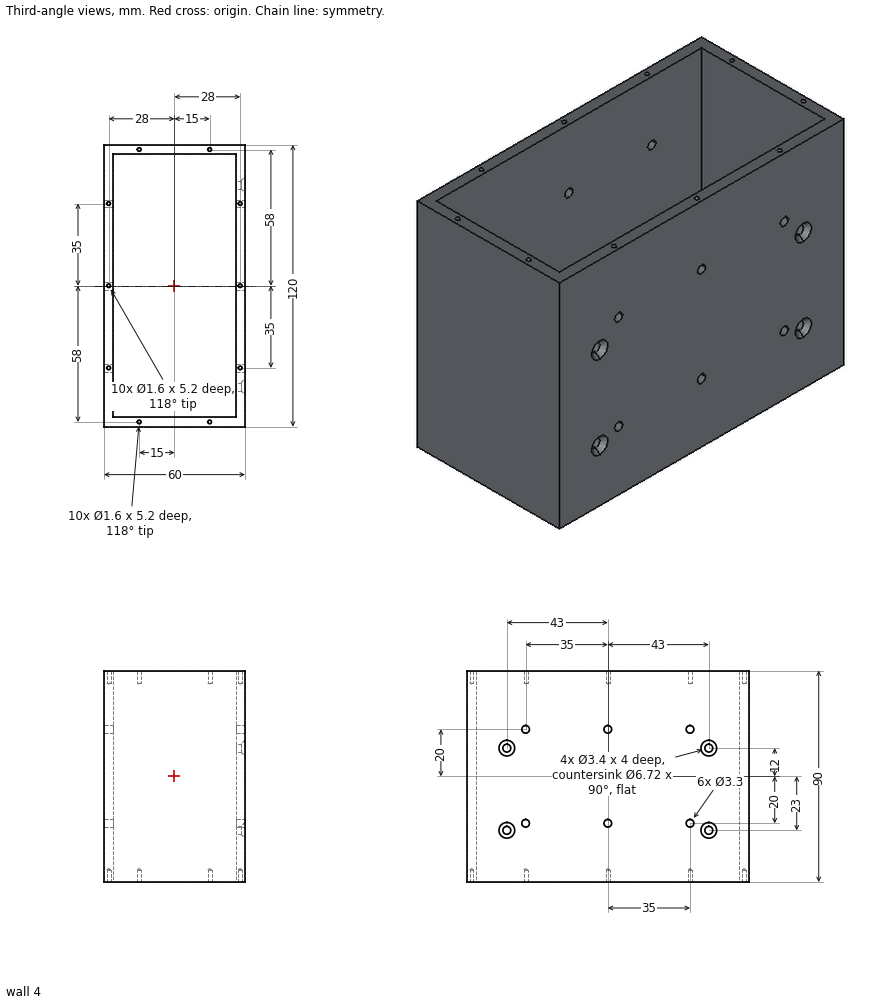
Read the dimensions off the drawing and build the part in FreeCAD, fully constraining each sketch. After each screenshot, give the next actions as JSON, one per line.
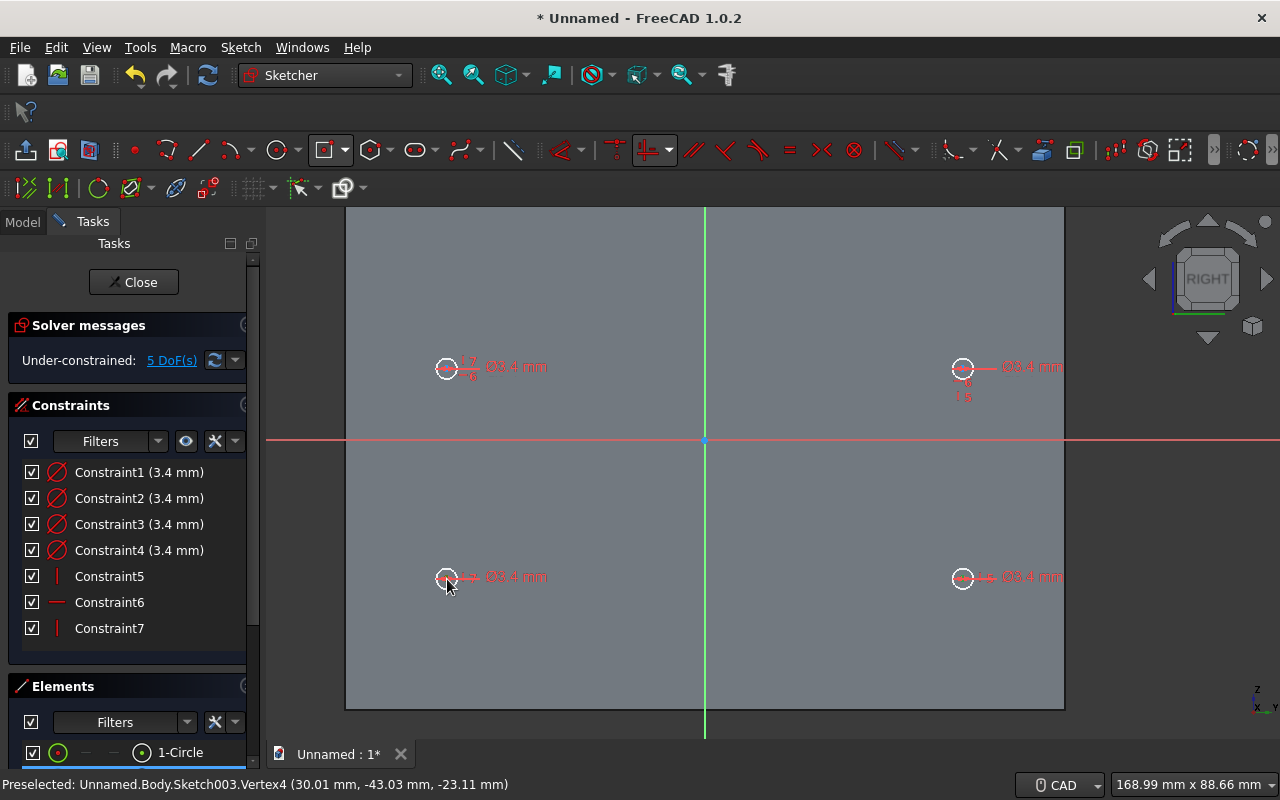
{"action": "left_click", "coordinate": [672, 150]}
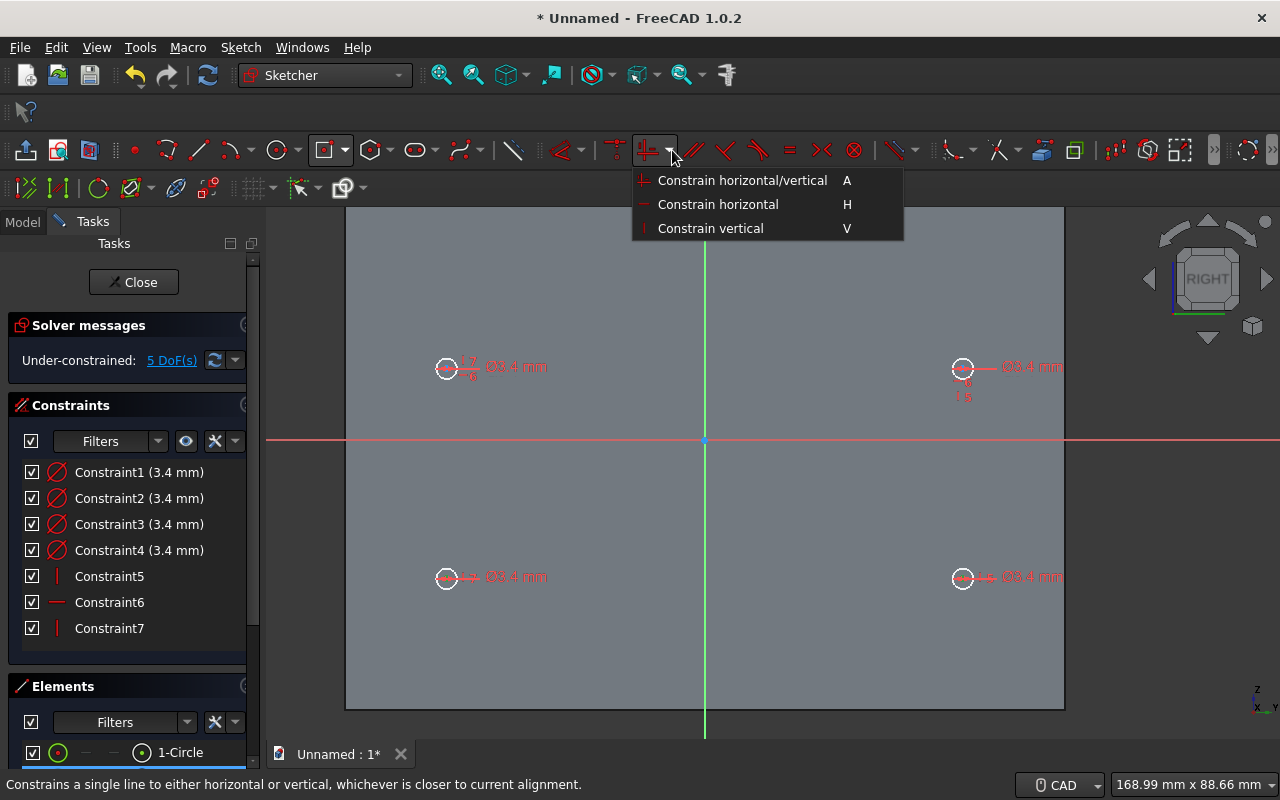
{"action": "left_click", "coordinate": [768, 204]}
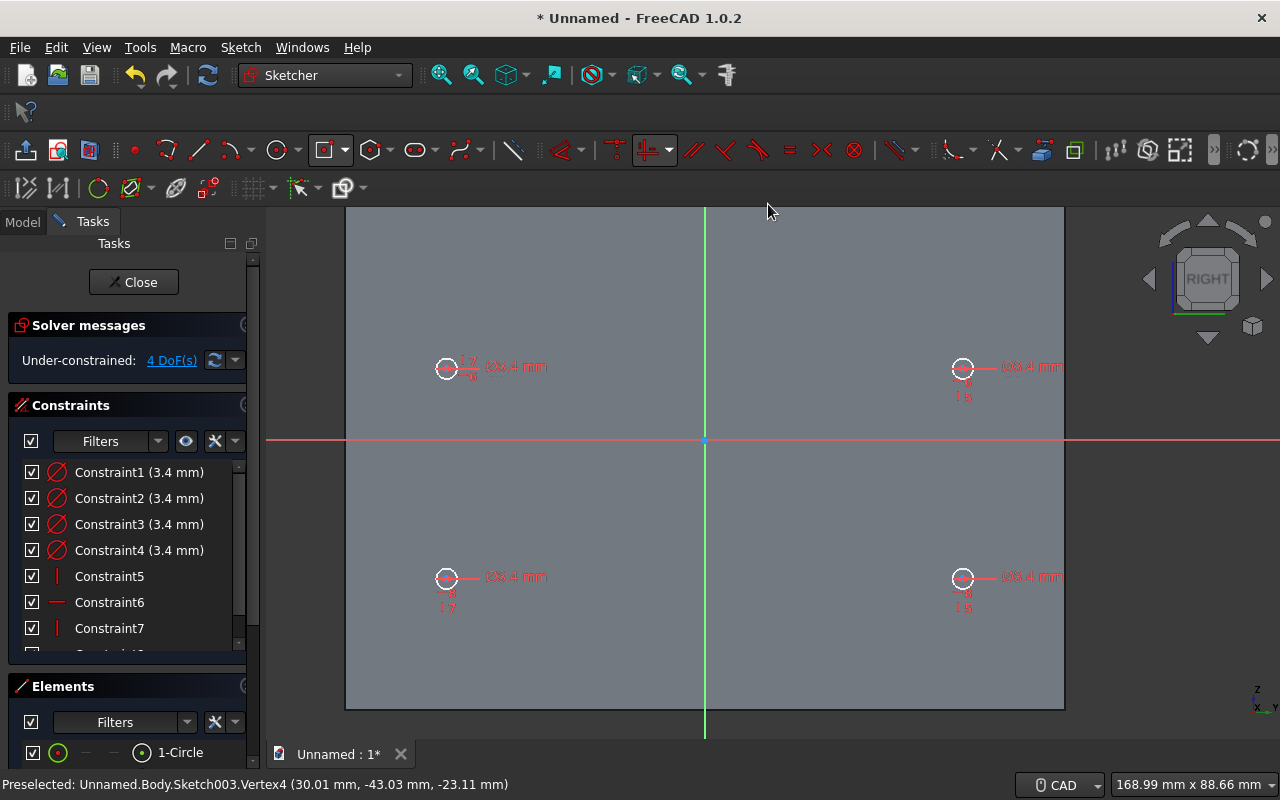
{"action": "left_click", "coordinate": [560, 150]}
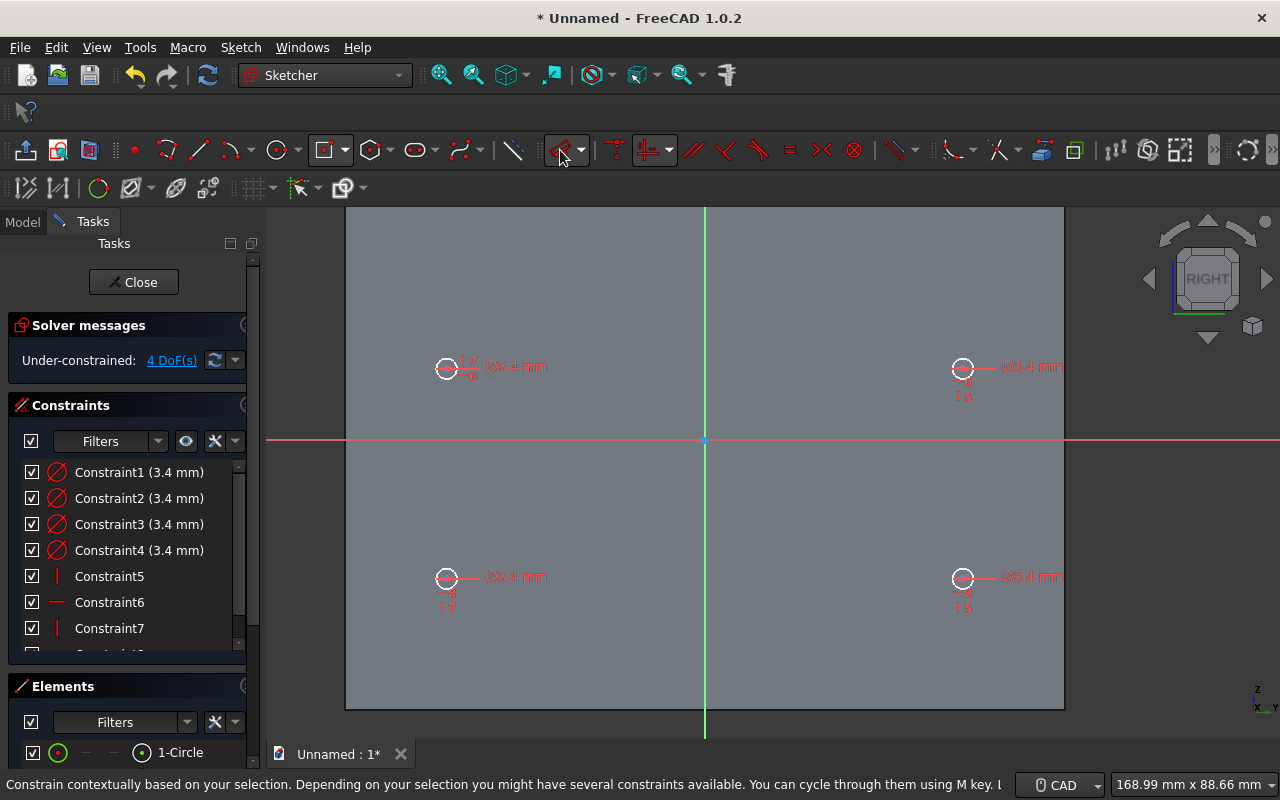
{"action": "left_click", "coordinate": [963, 369]}
{"action": "left_click", "coordinate": [834, 335]}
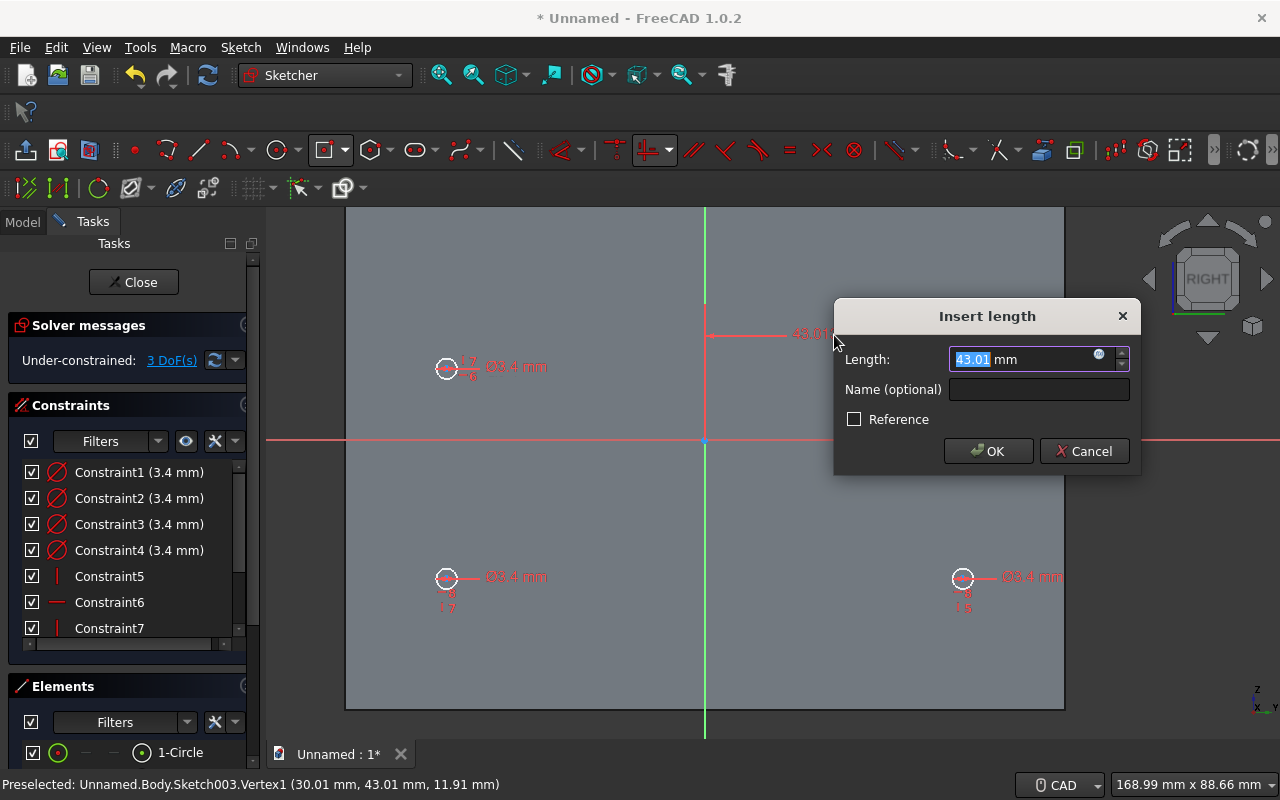
{"action": "type", "text": "43"}
{"action": "key", "text": "Return"}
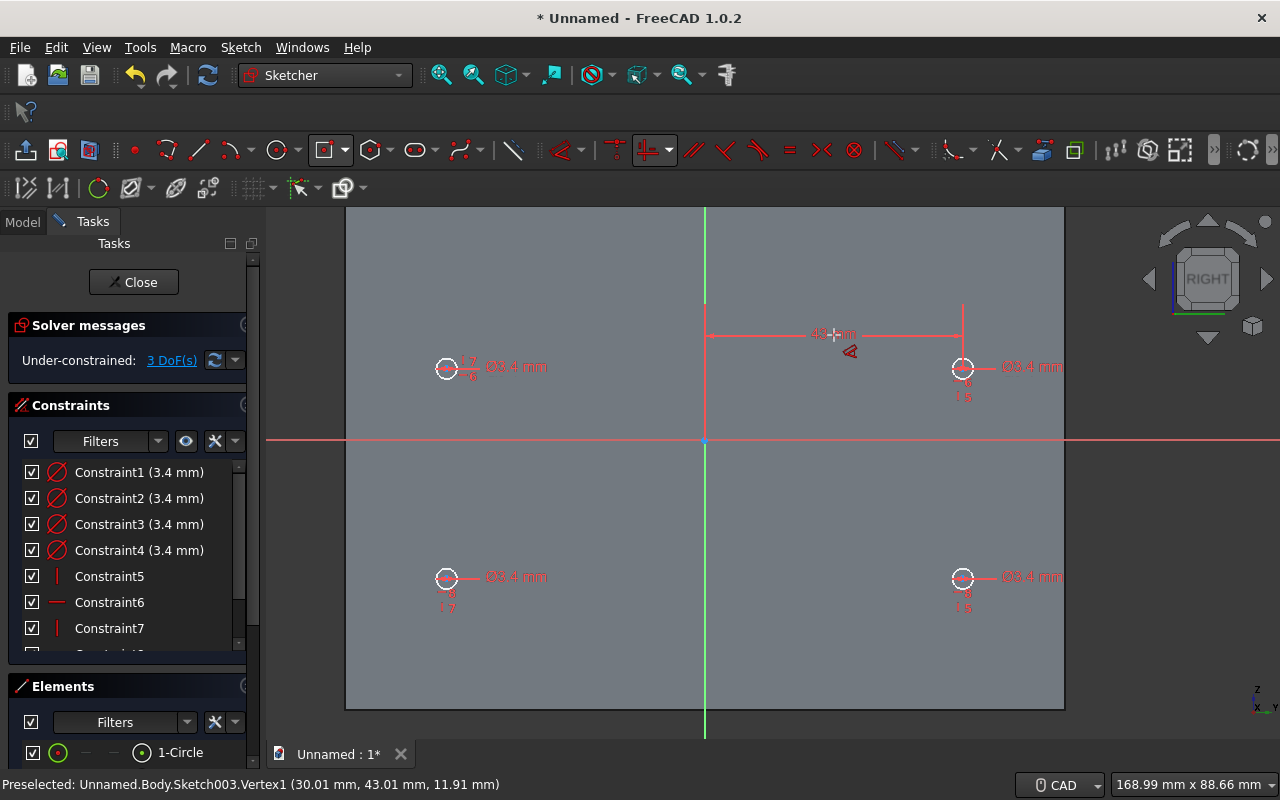
{"action": "left_click", "coordinate": [963, 369]}
{"action": "left_click", "coordinate": [997, 404]}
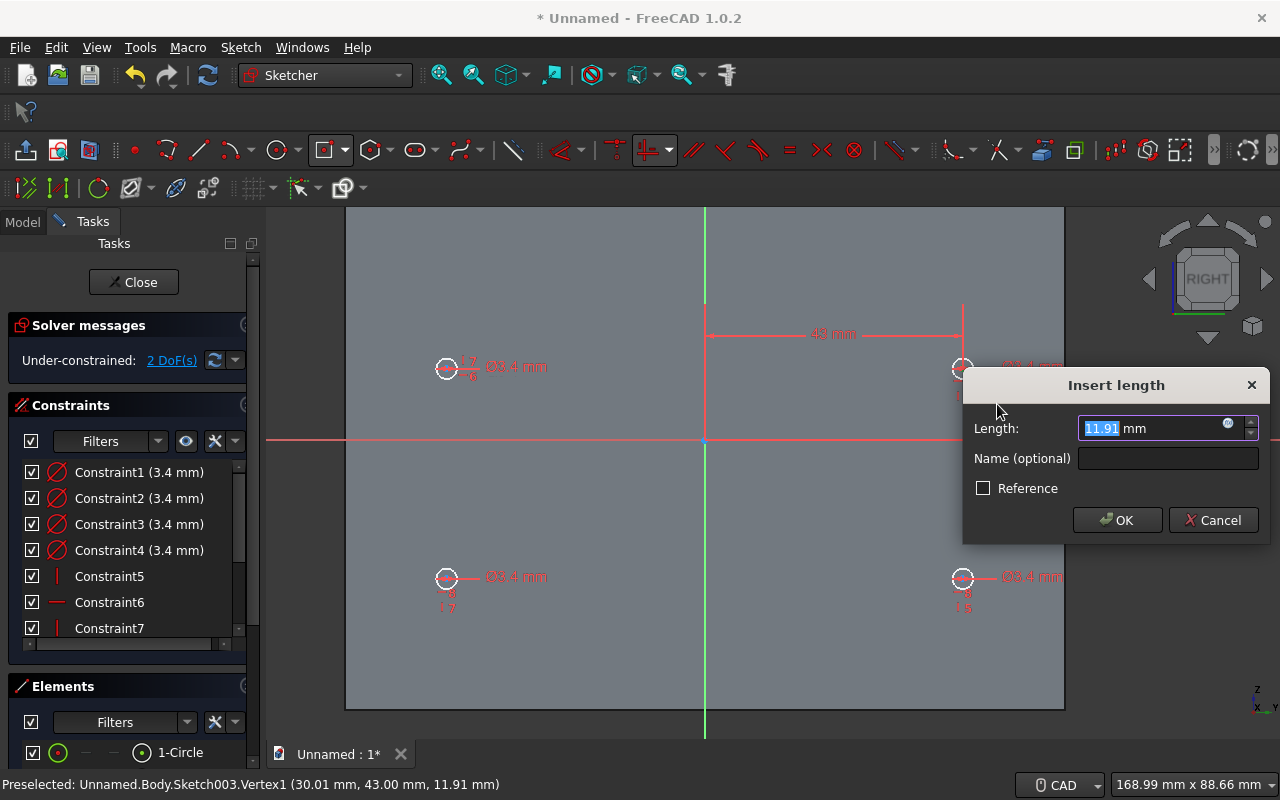
{"action": "type", "text": "12"}
{"action": "key", "text": "Return"}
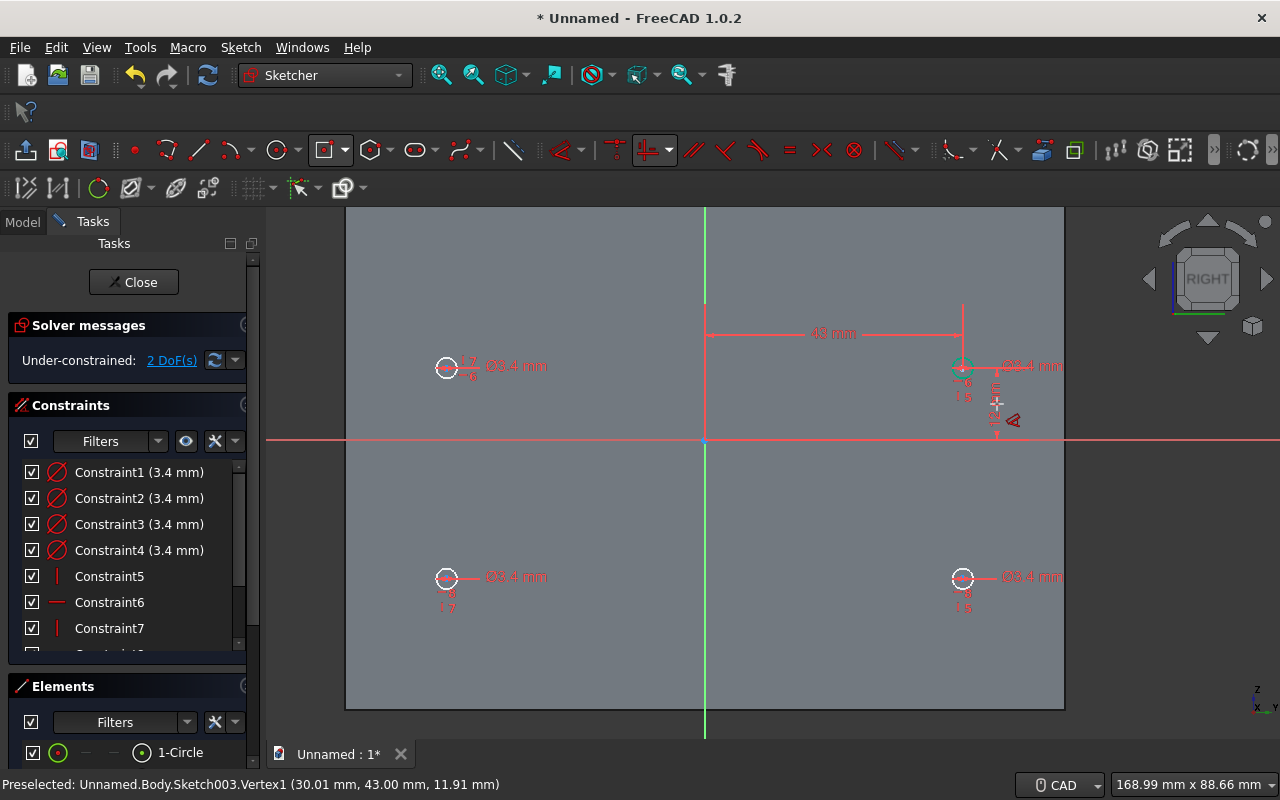
{"action": "left_click", "coordinate": [963, 579]}
{"action": "left_click", "coordinate": [997, 510]}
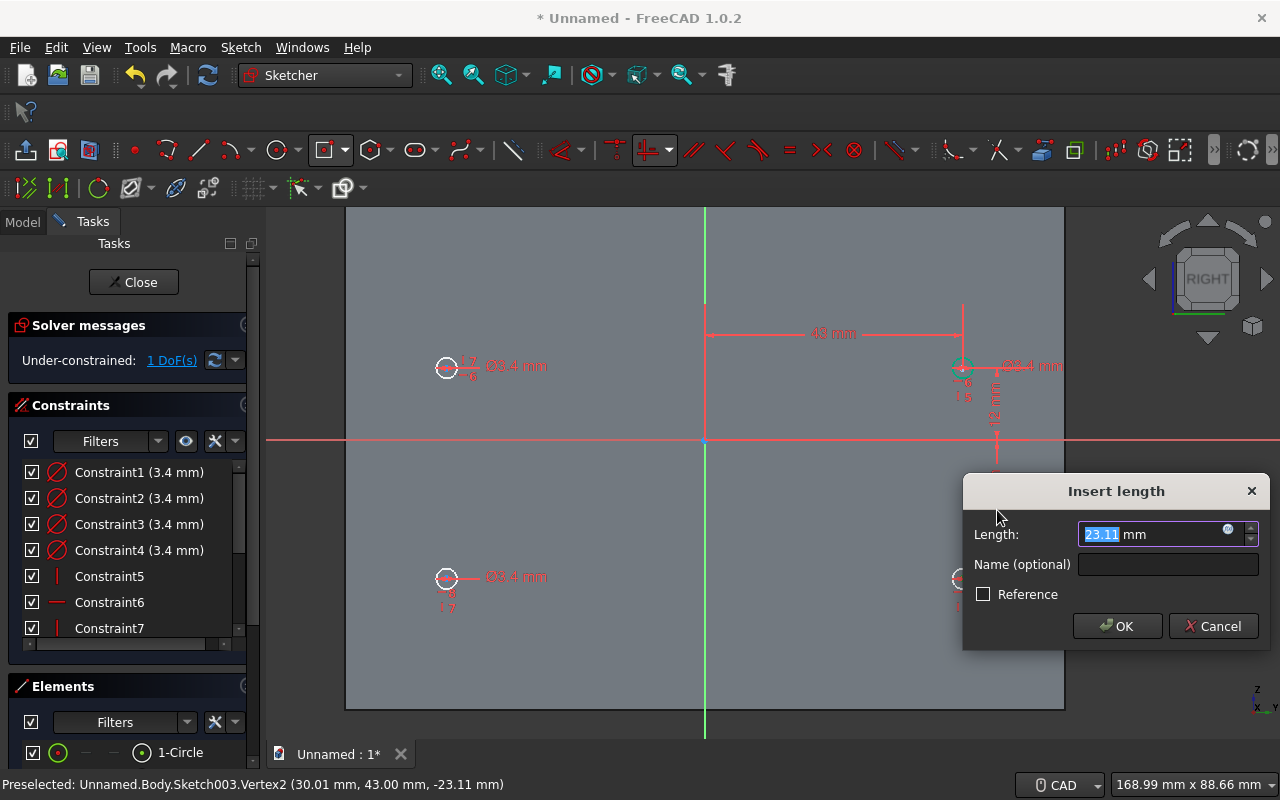
{"action": "type", "text": "23"}
{"action": "key", "text": "Return"}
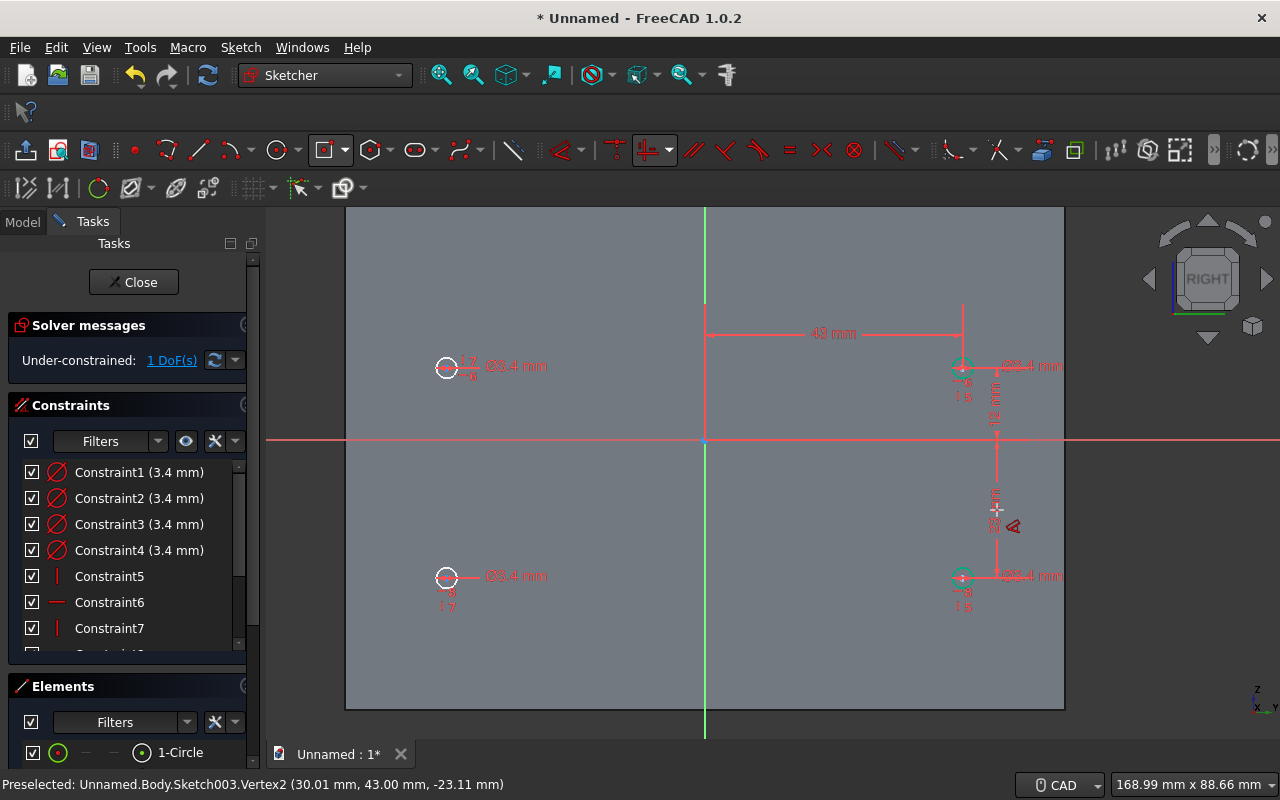
{"action": "left_click", "coordinate": [447, 368]}
{"action": "left_click", "coordinate": [576, 334]}